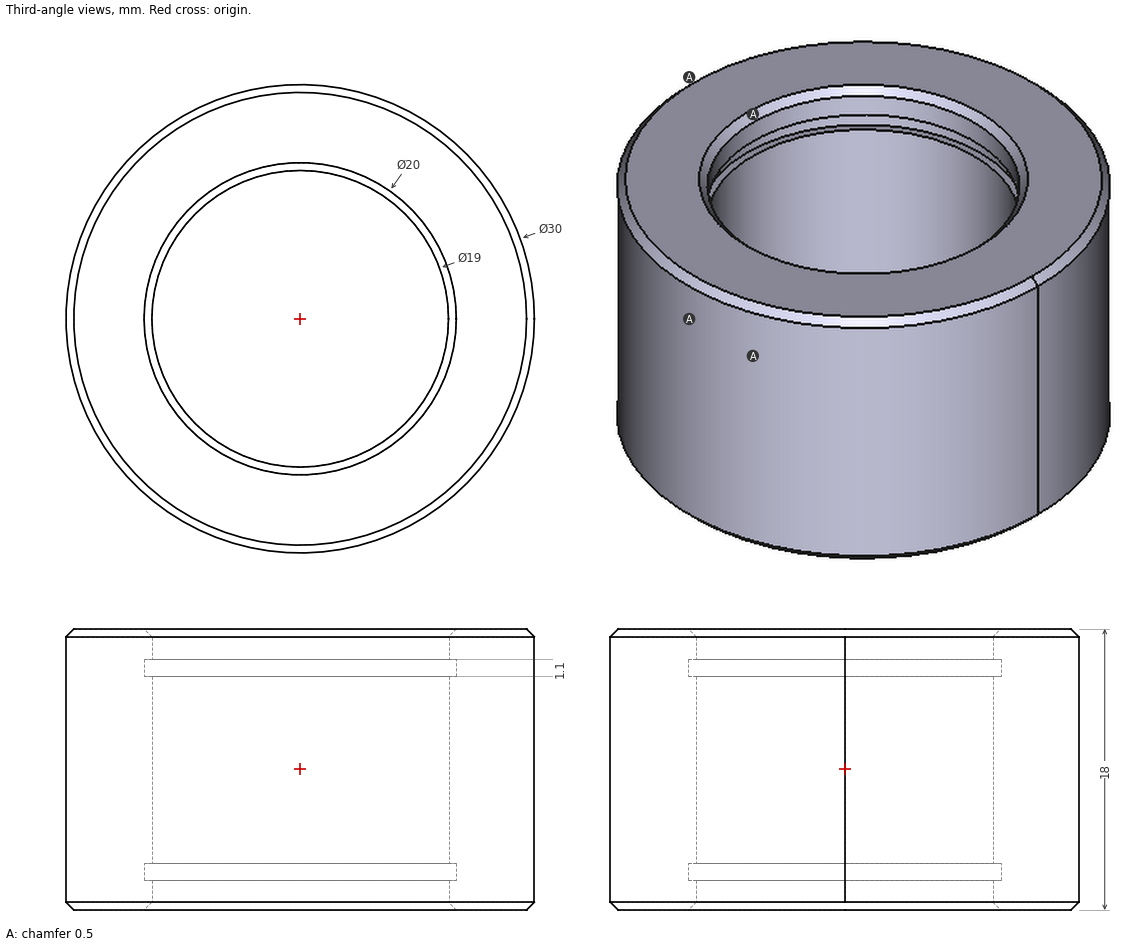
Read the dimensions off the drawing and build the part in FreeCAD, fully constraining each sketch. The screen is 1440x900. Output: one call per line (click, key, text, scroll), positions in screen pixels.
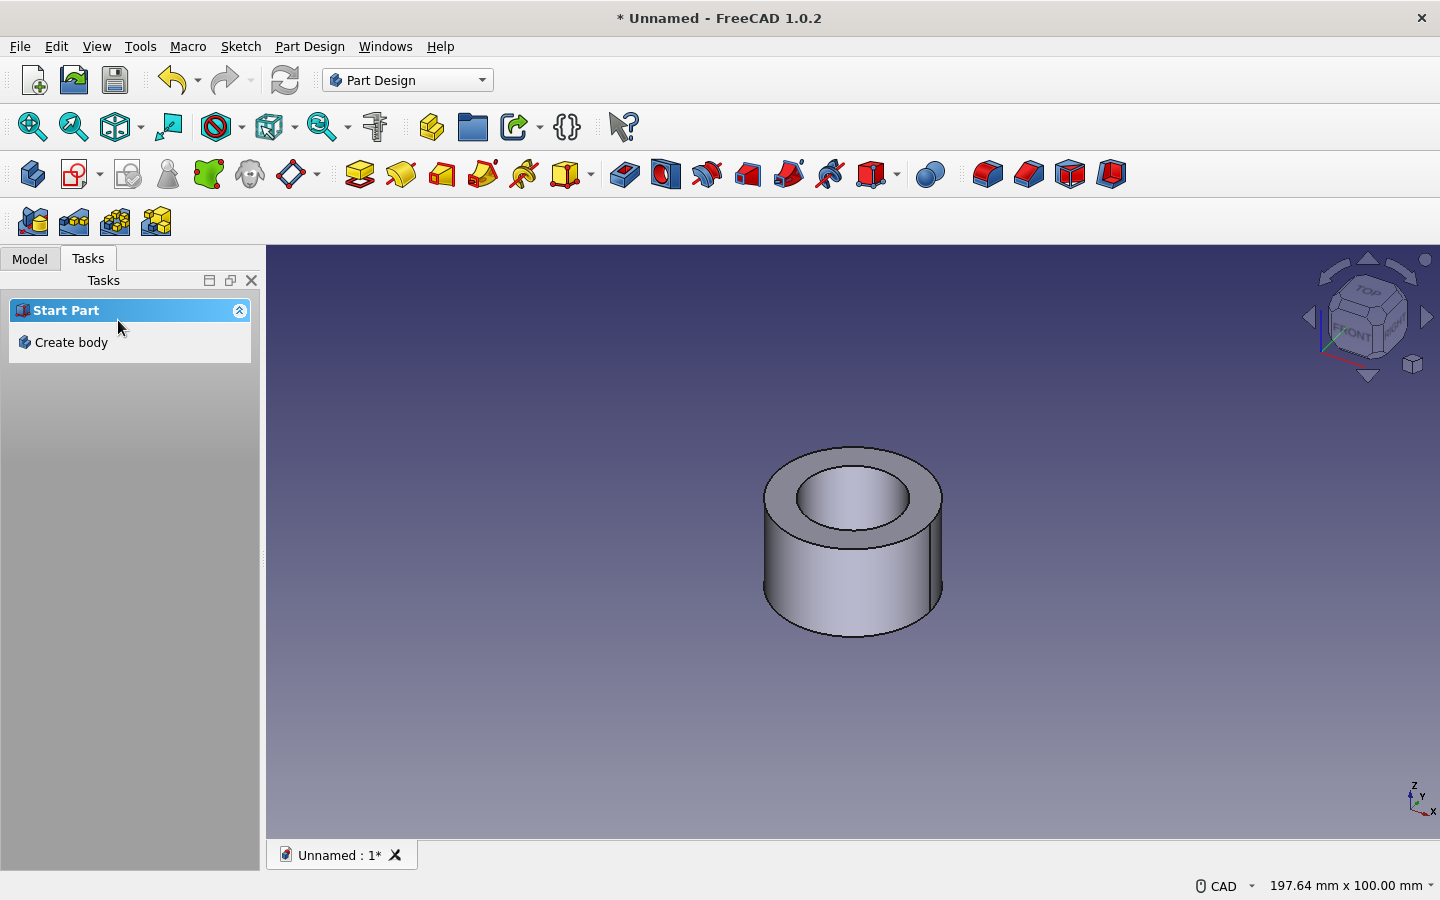
click(33, 128)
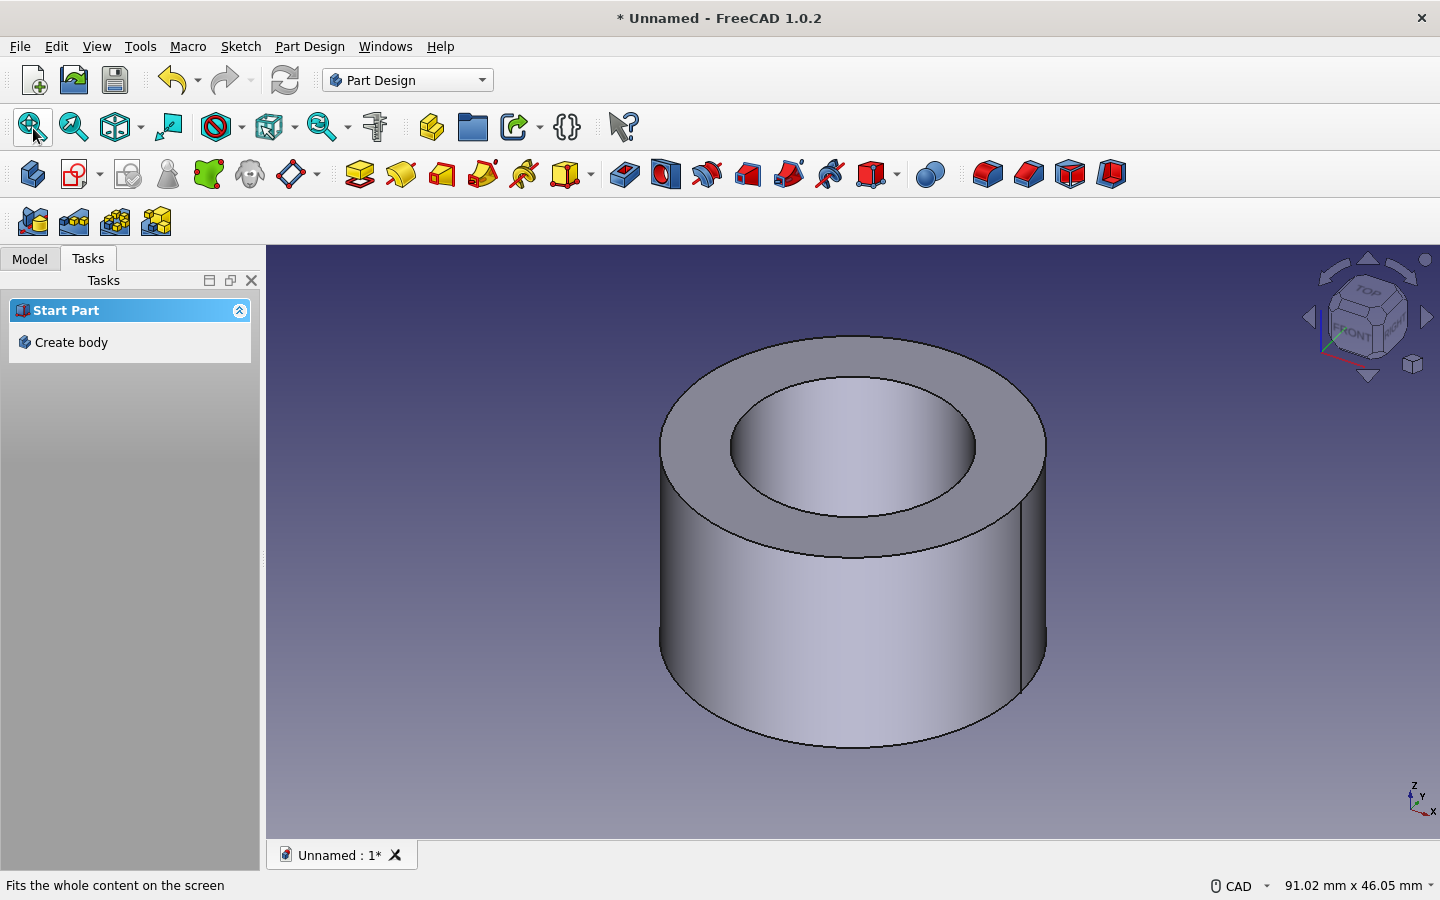
click(30, 258)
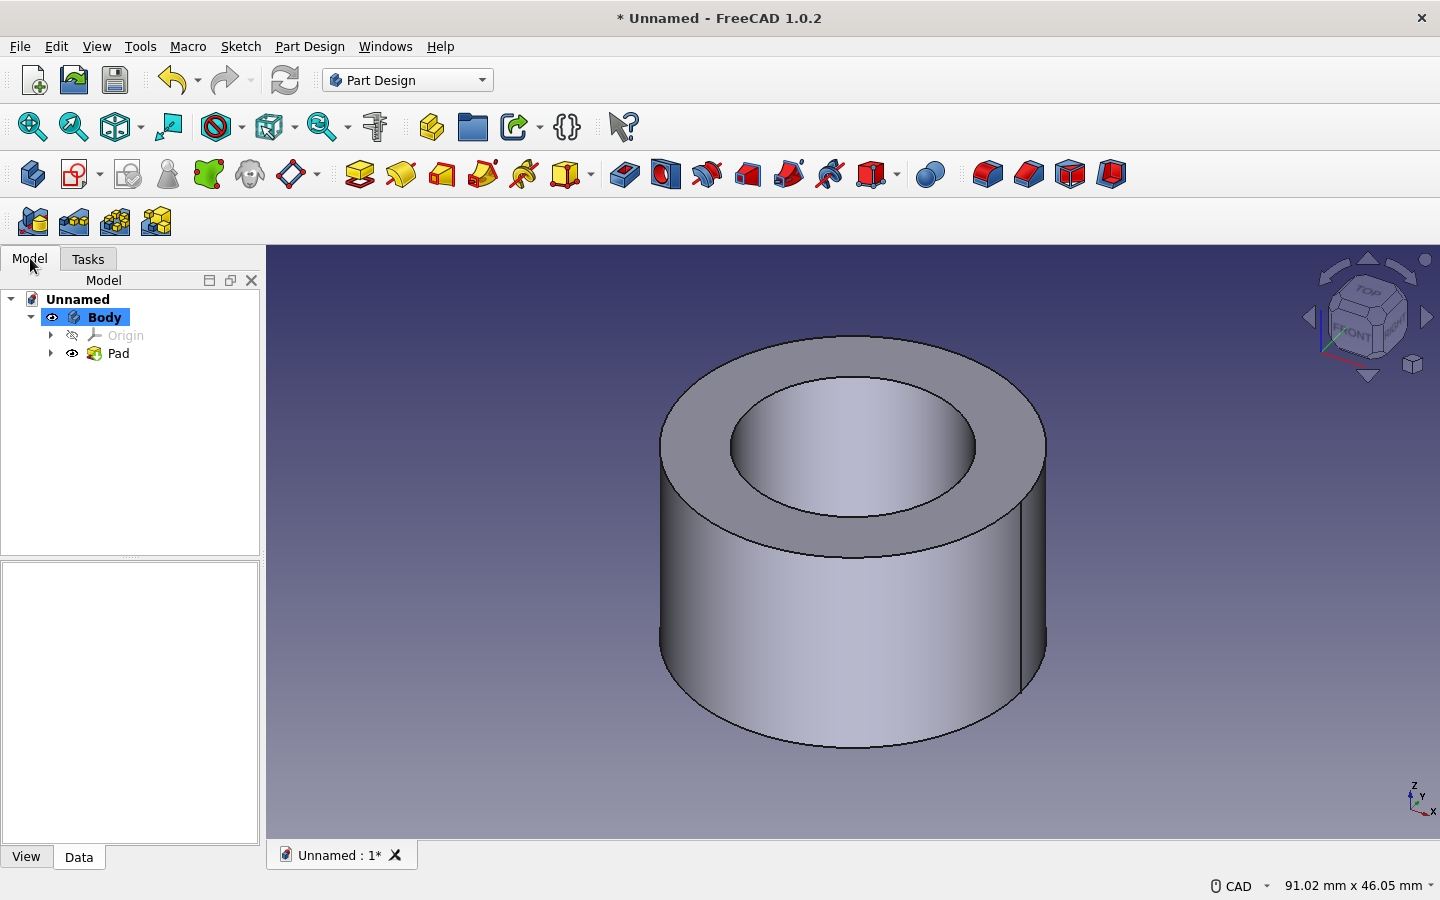
click(51, 335)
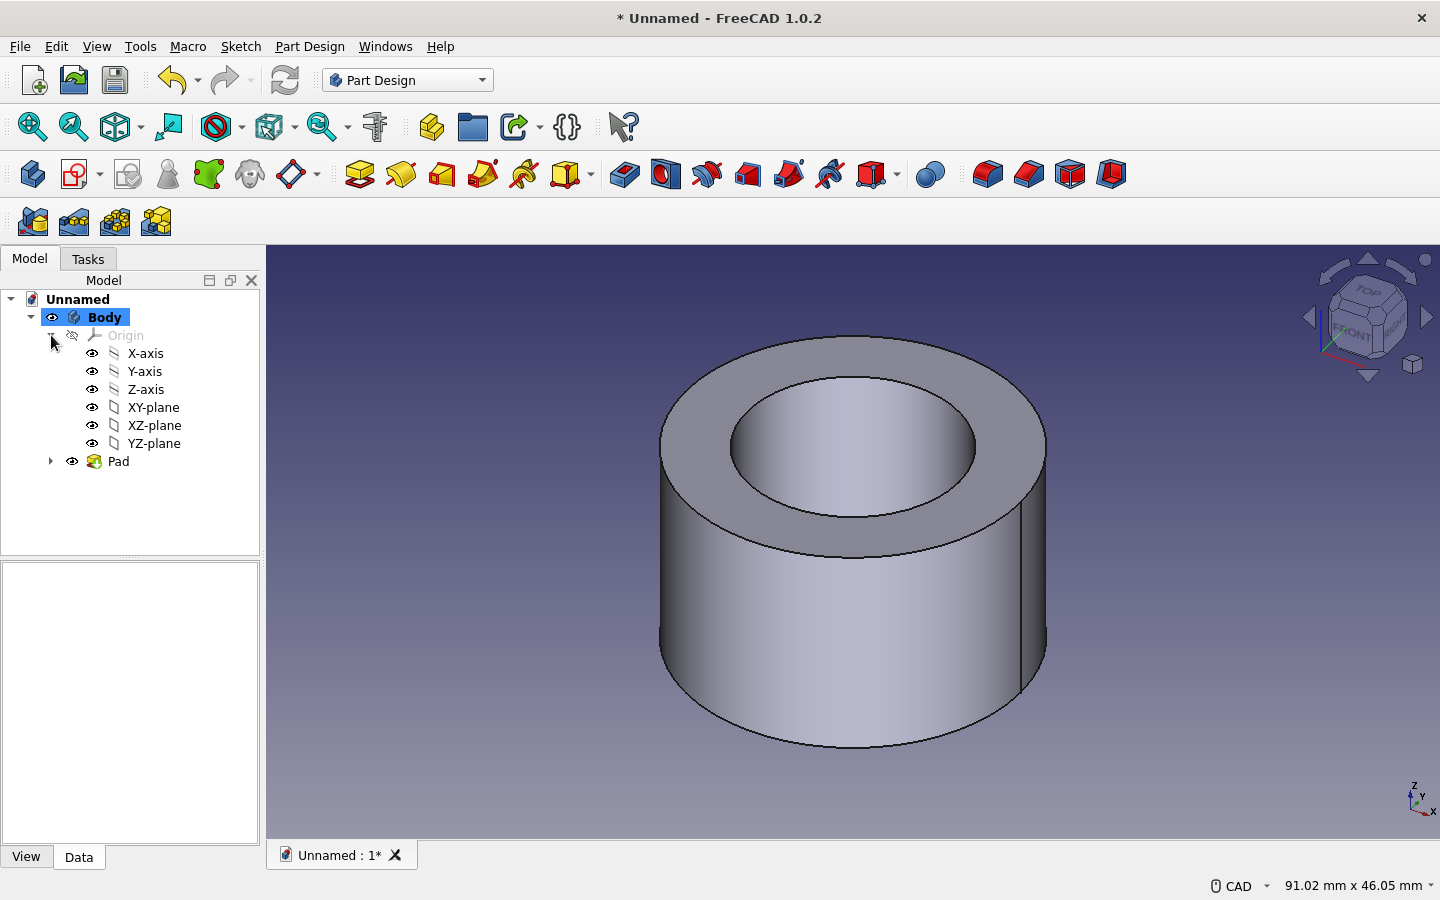
click(137, 407)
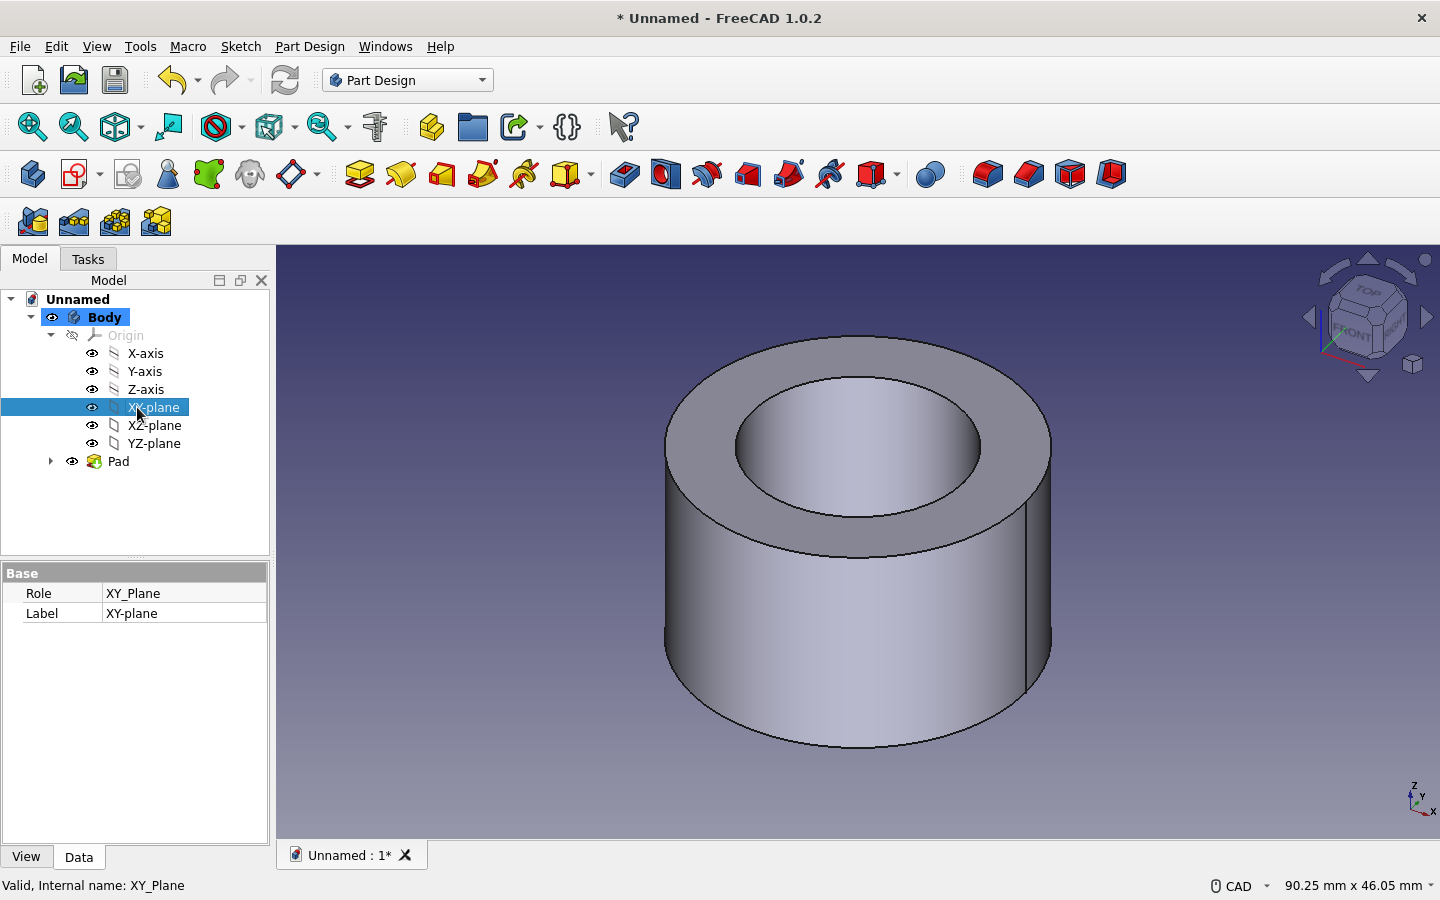
click(290, 174)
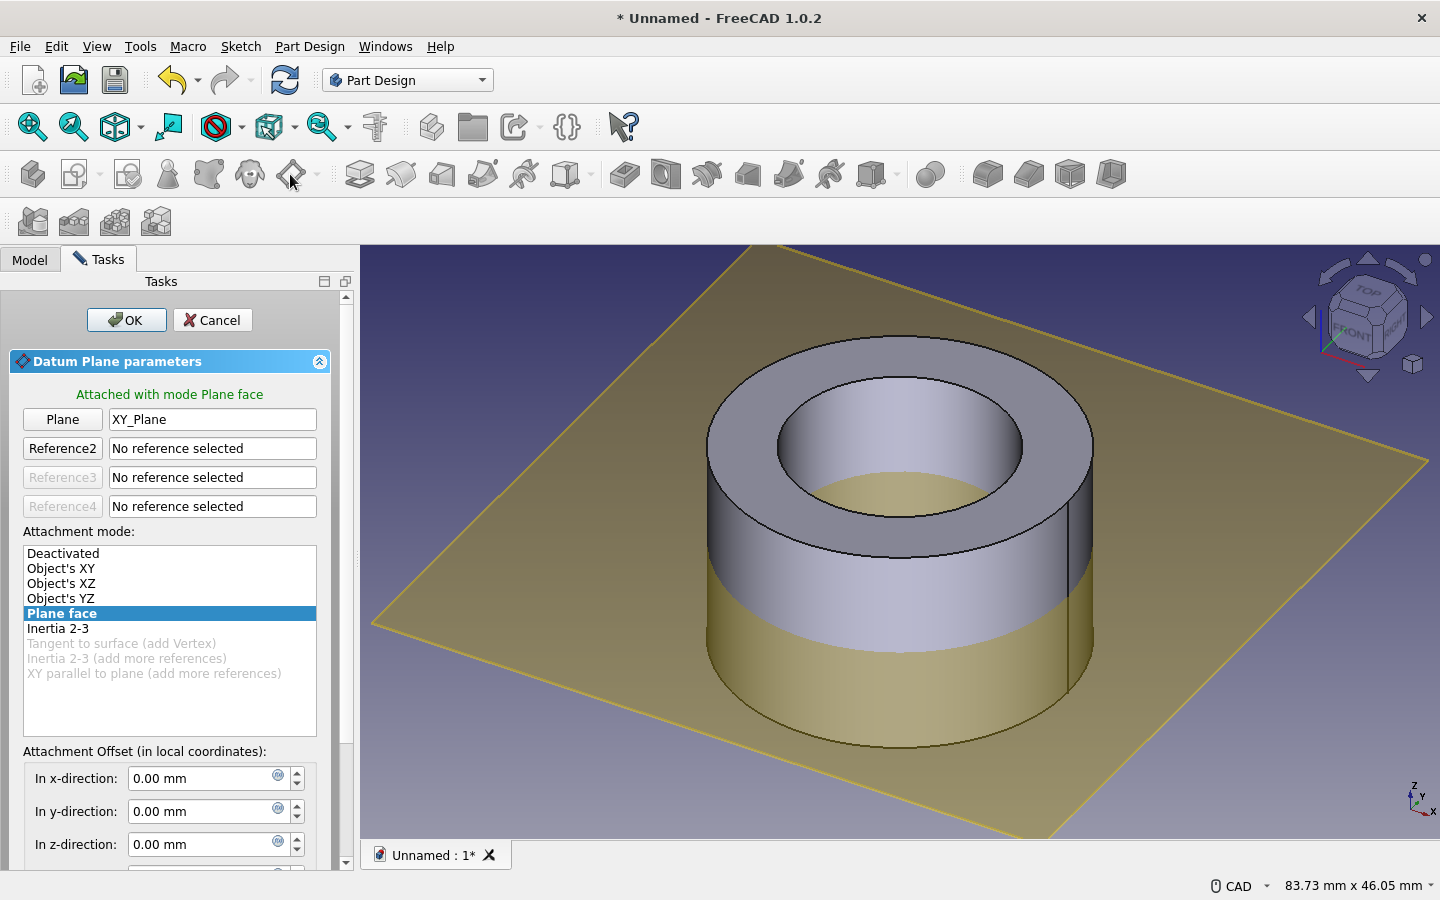
triple_click(210, 844)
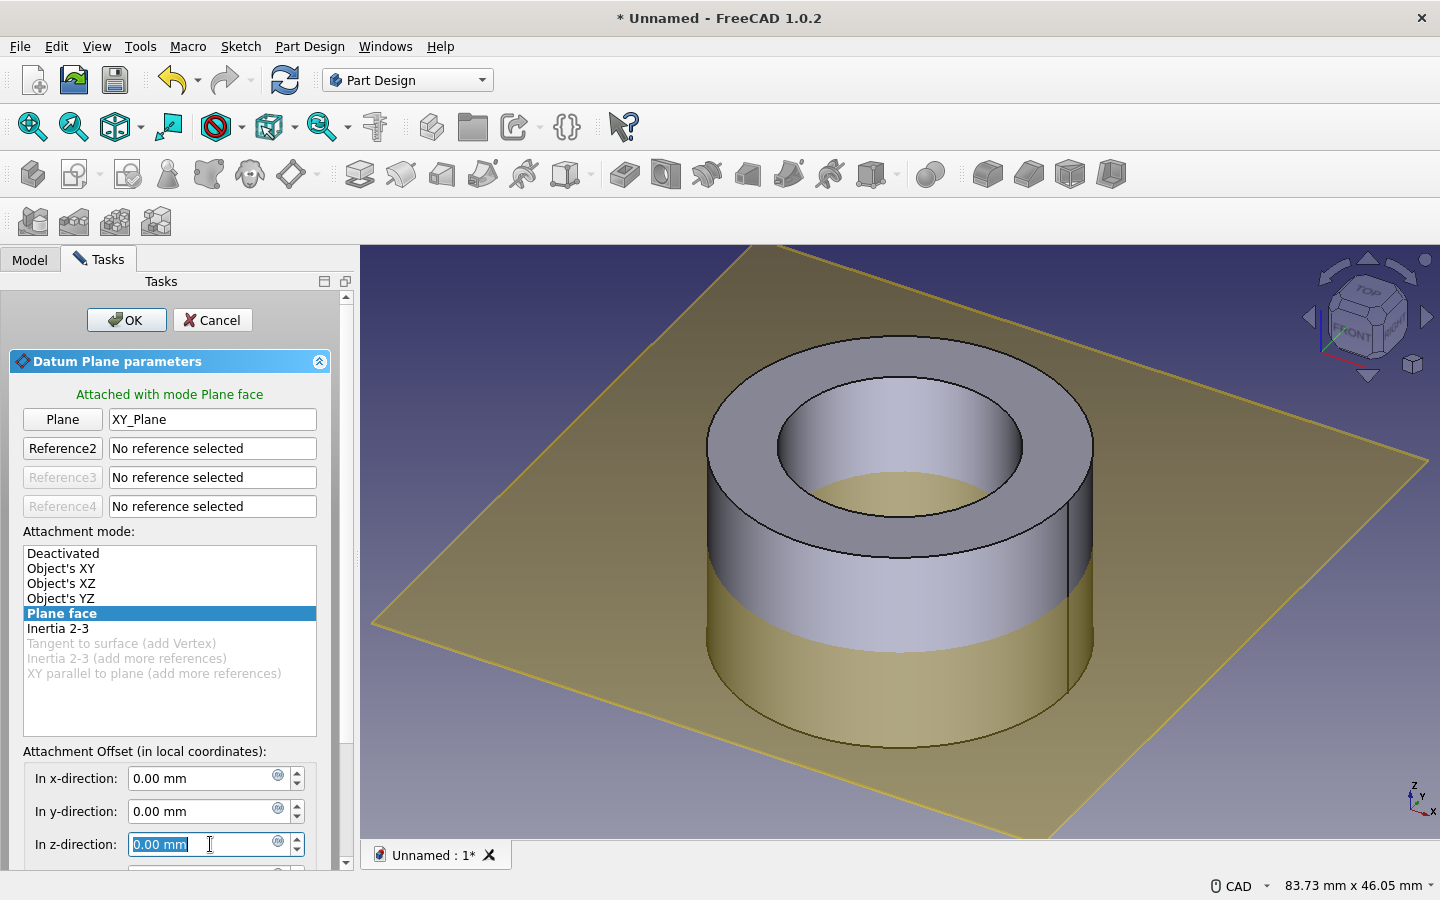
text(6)
key(Tab)